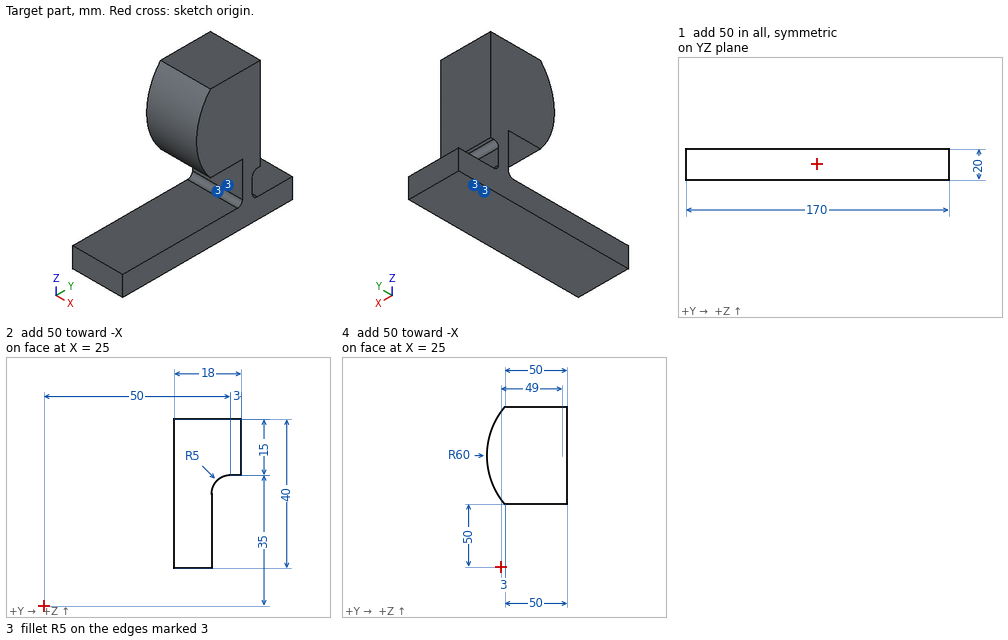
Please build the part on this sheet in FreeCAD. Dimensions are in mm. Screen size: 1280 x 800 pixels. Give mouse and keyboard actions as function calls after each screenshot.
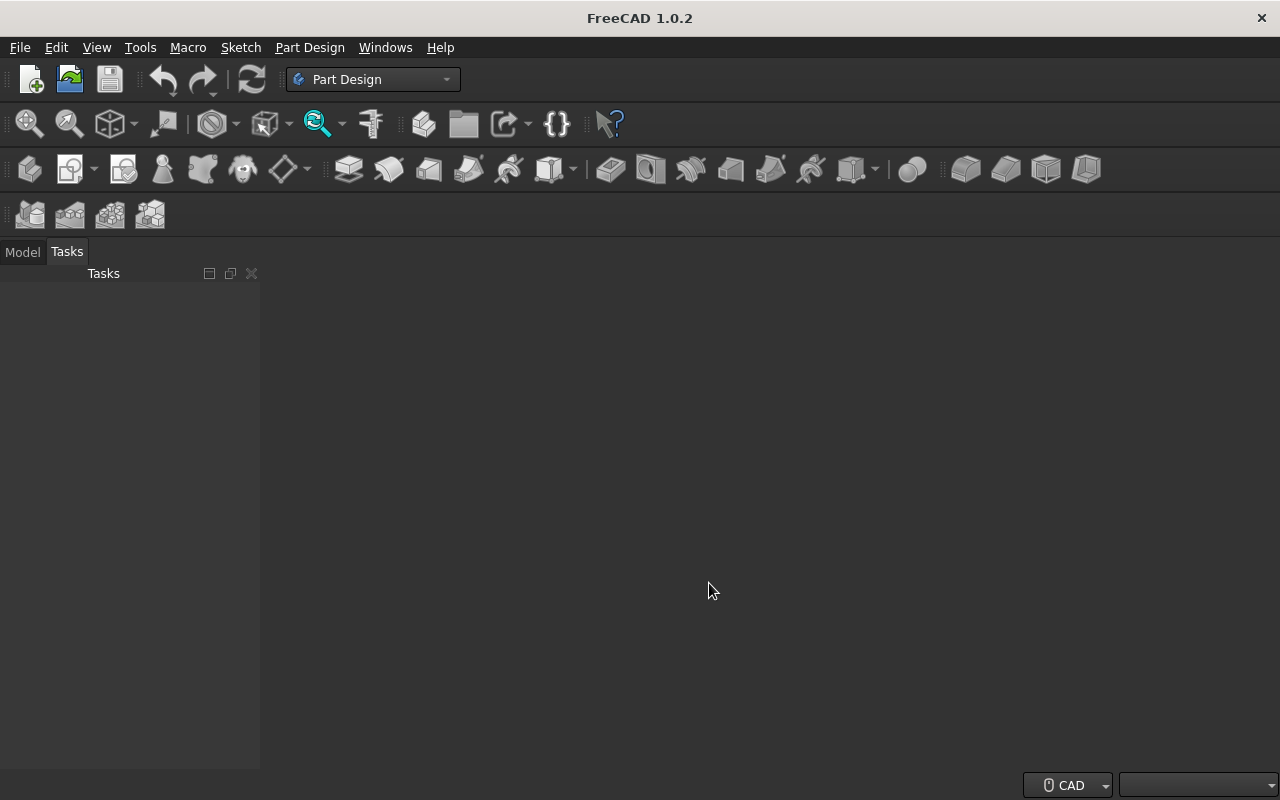
click(30, 80)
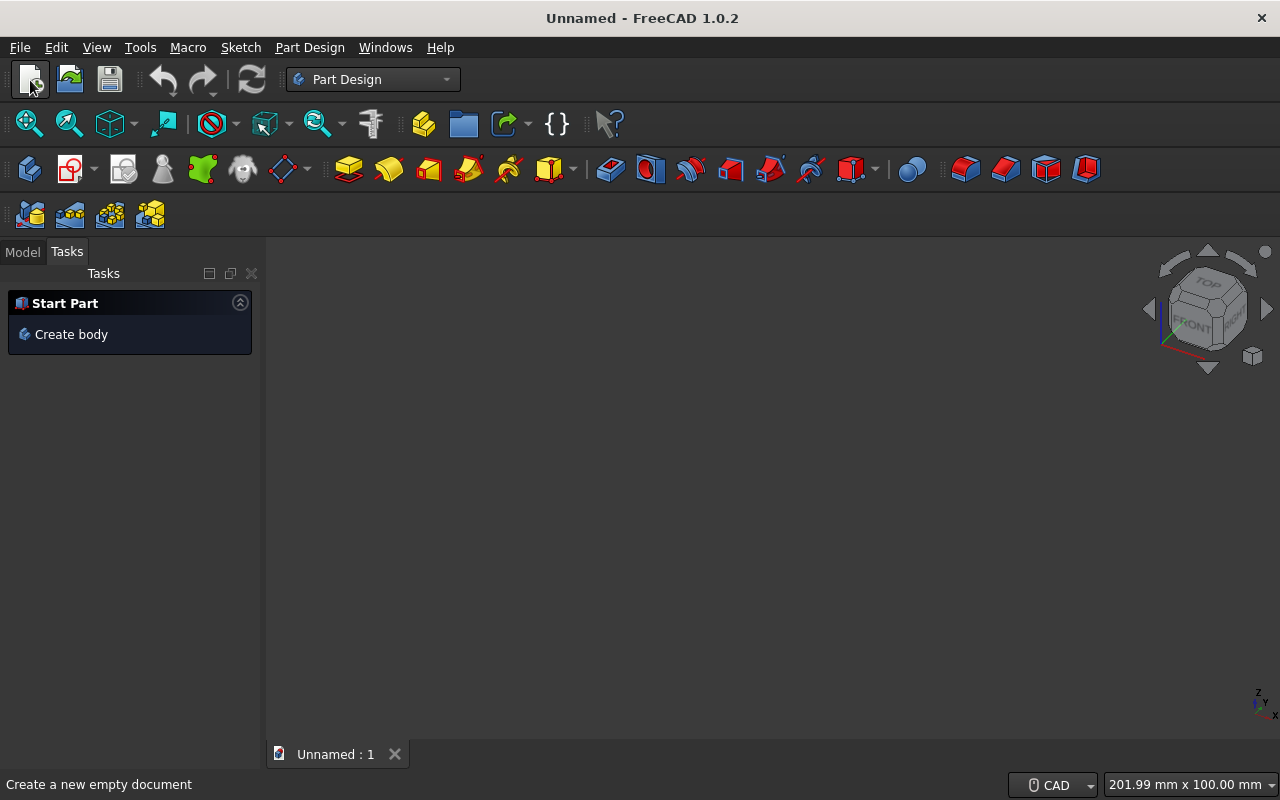
click(70, 170)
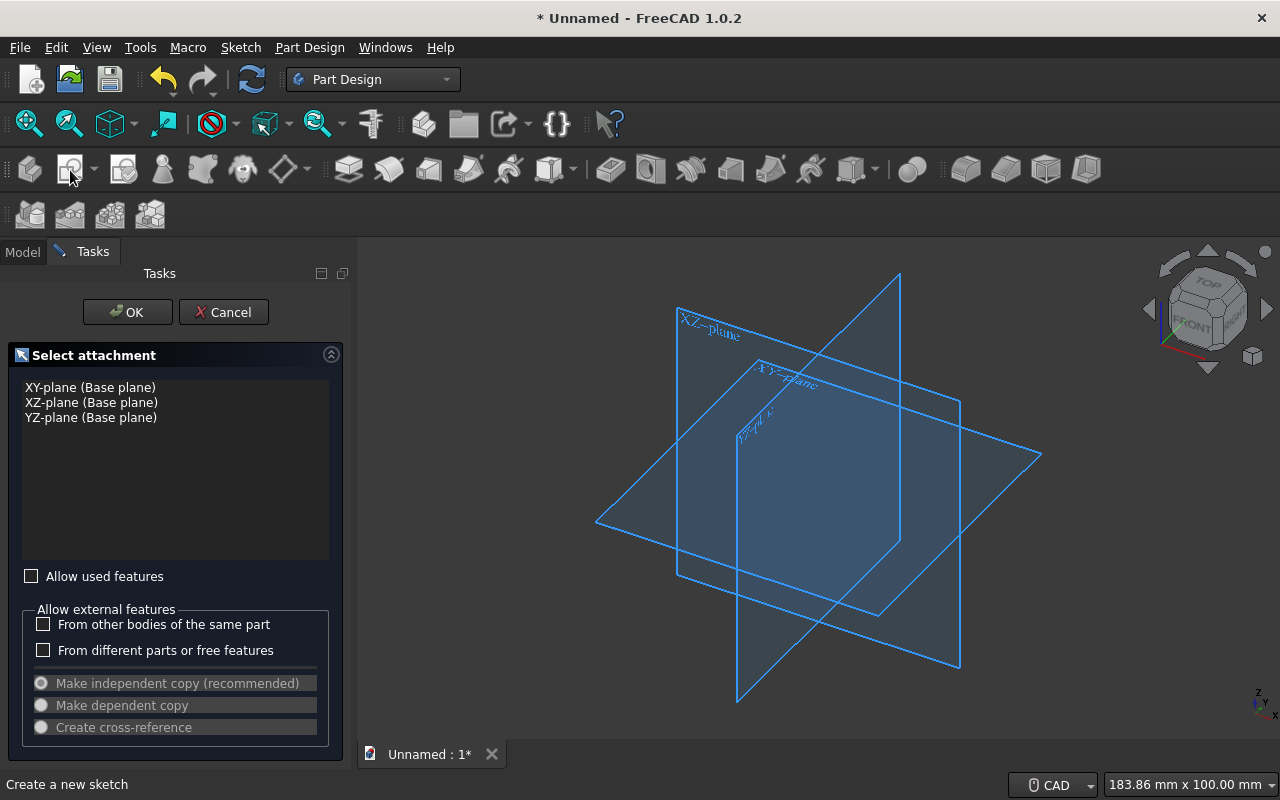
click(82, 418)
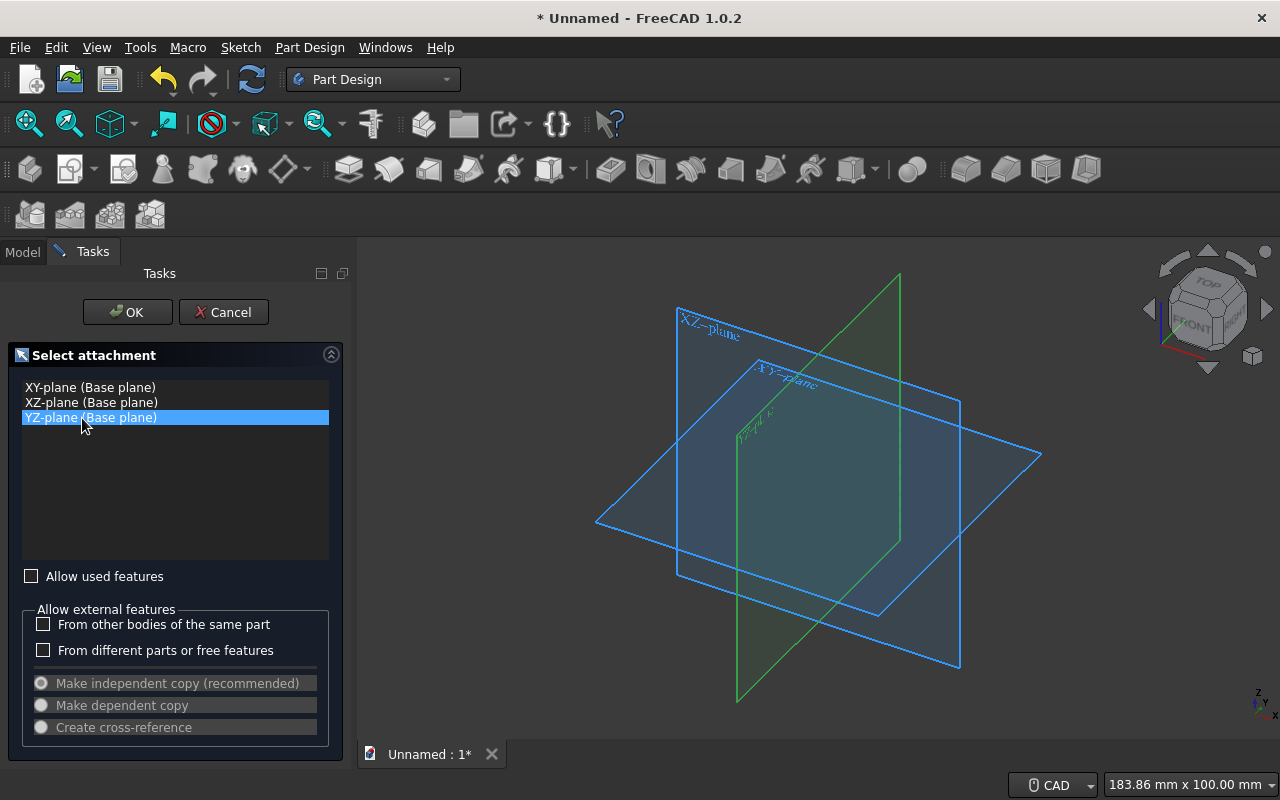
click(128, 312)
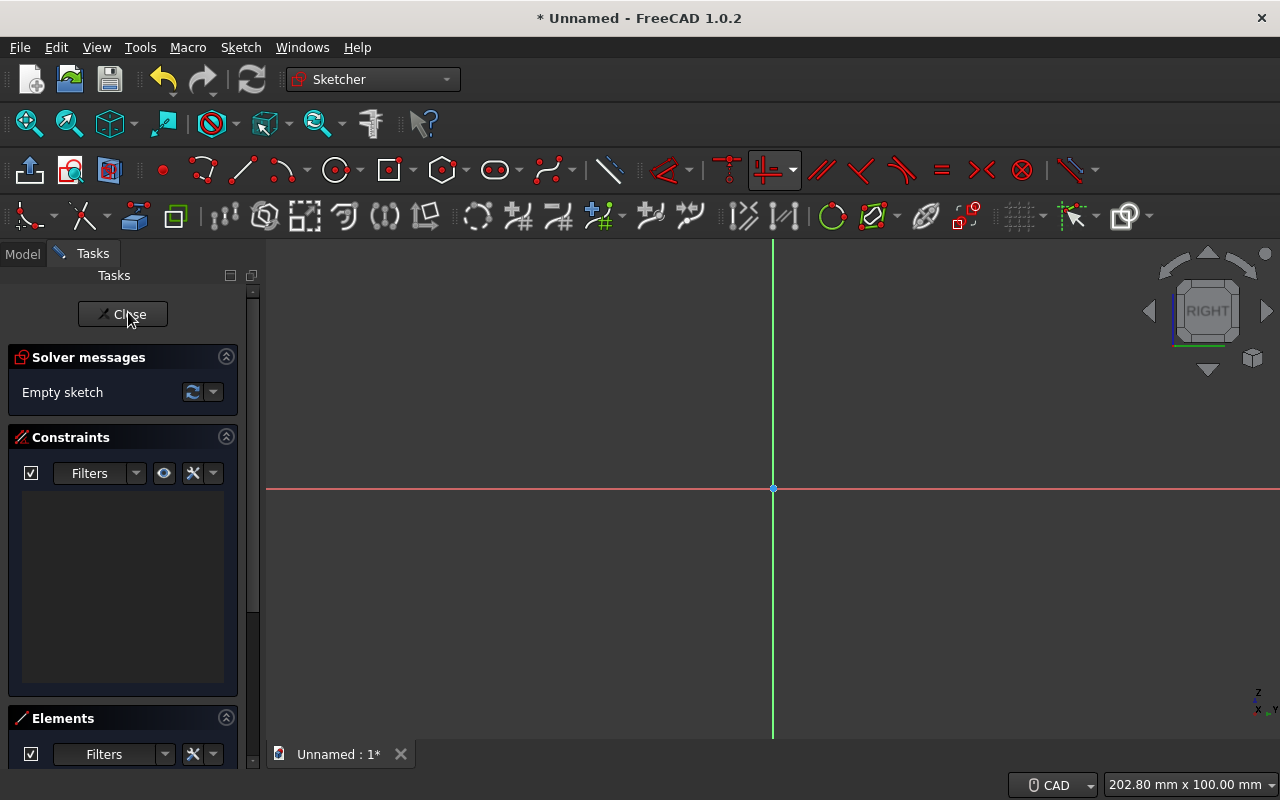
scroll(565, 489, down, 2)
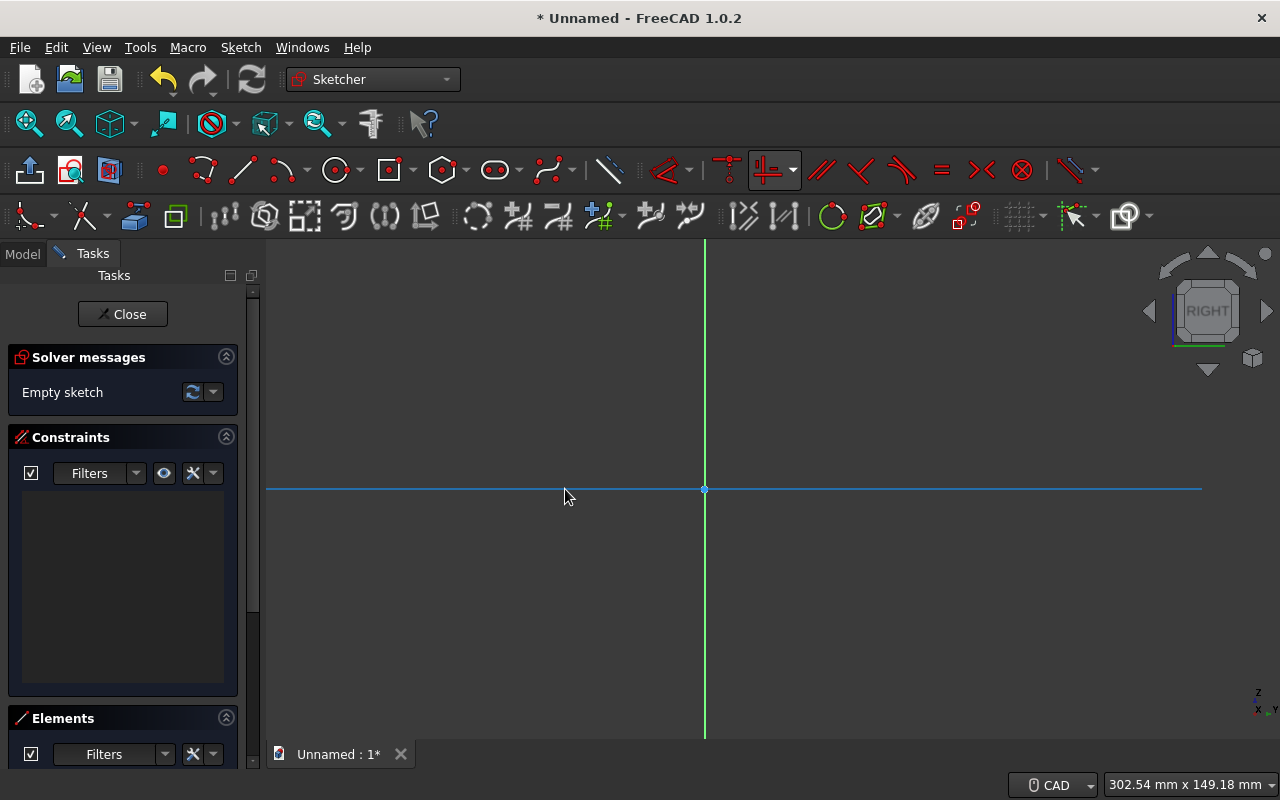
key(g)
key(v)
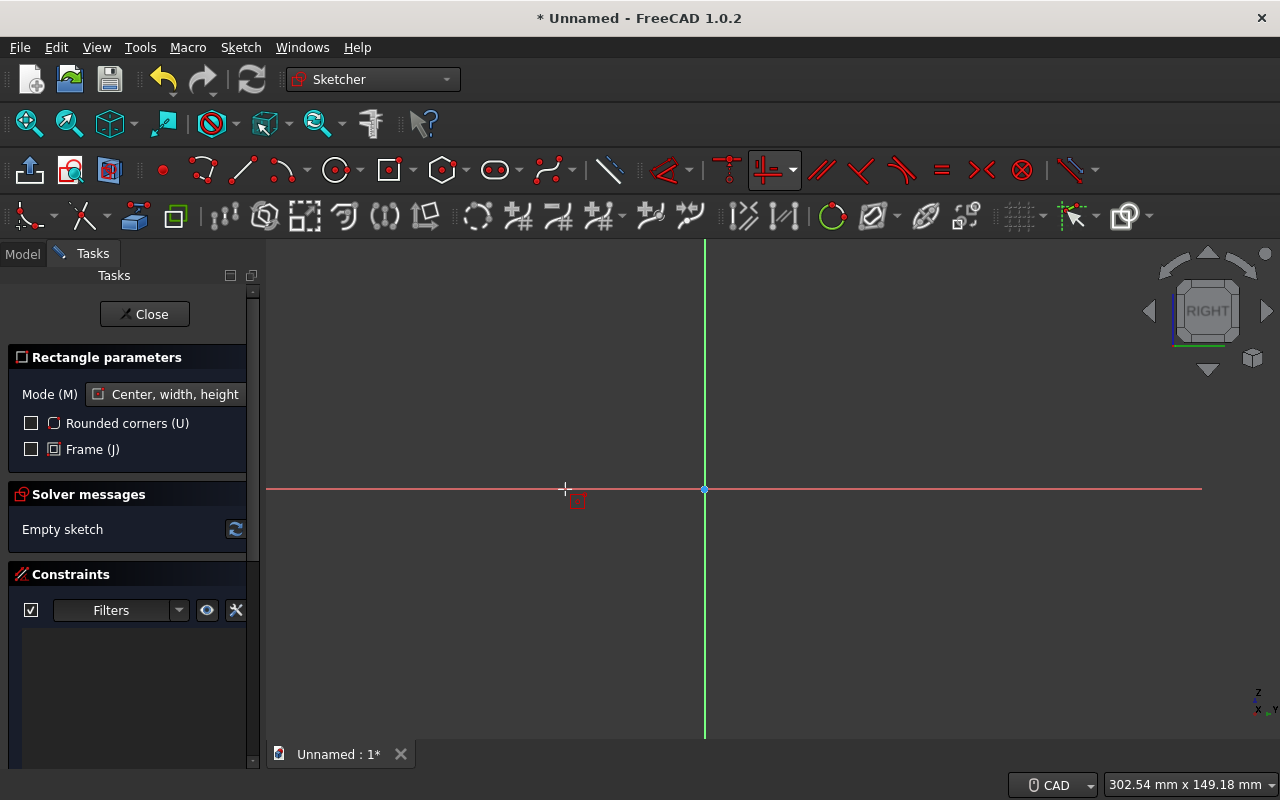
click(705, 489)
click(989, 456)
key(Escape)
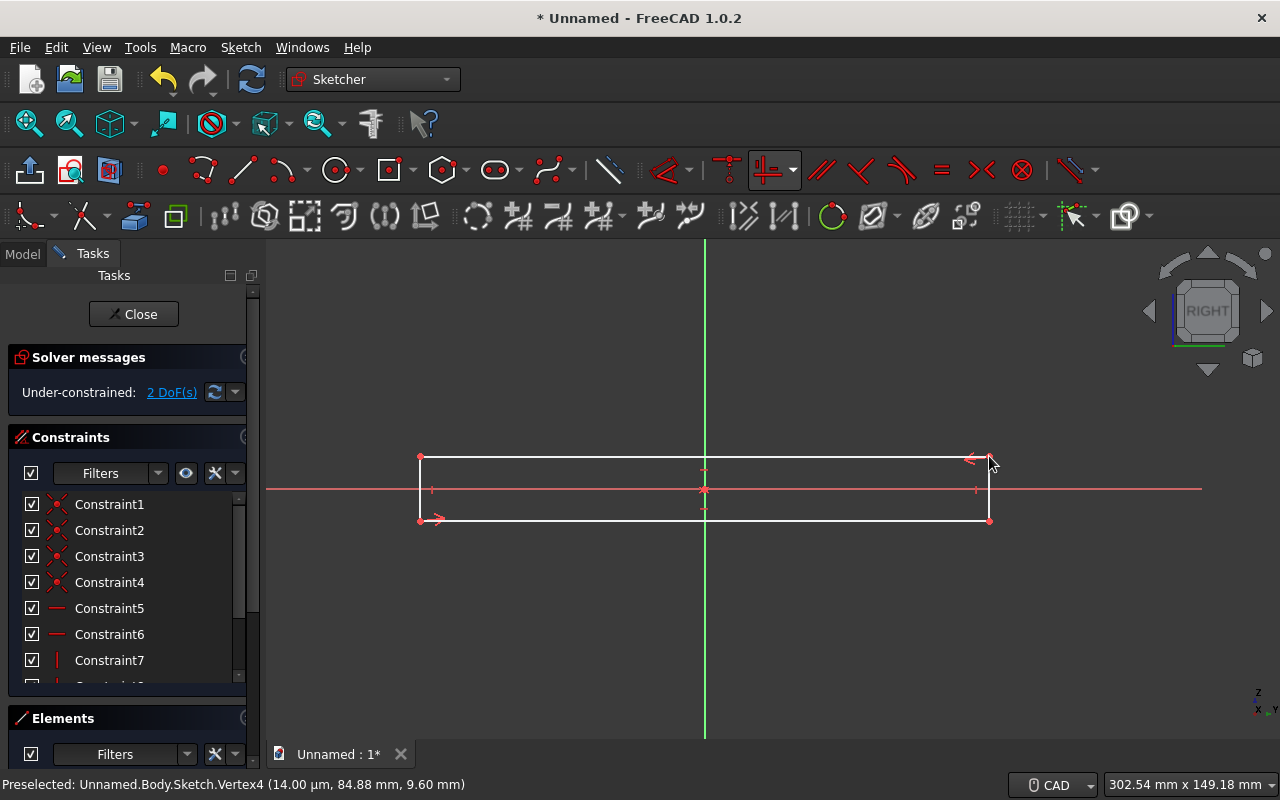
key(d)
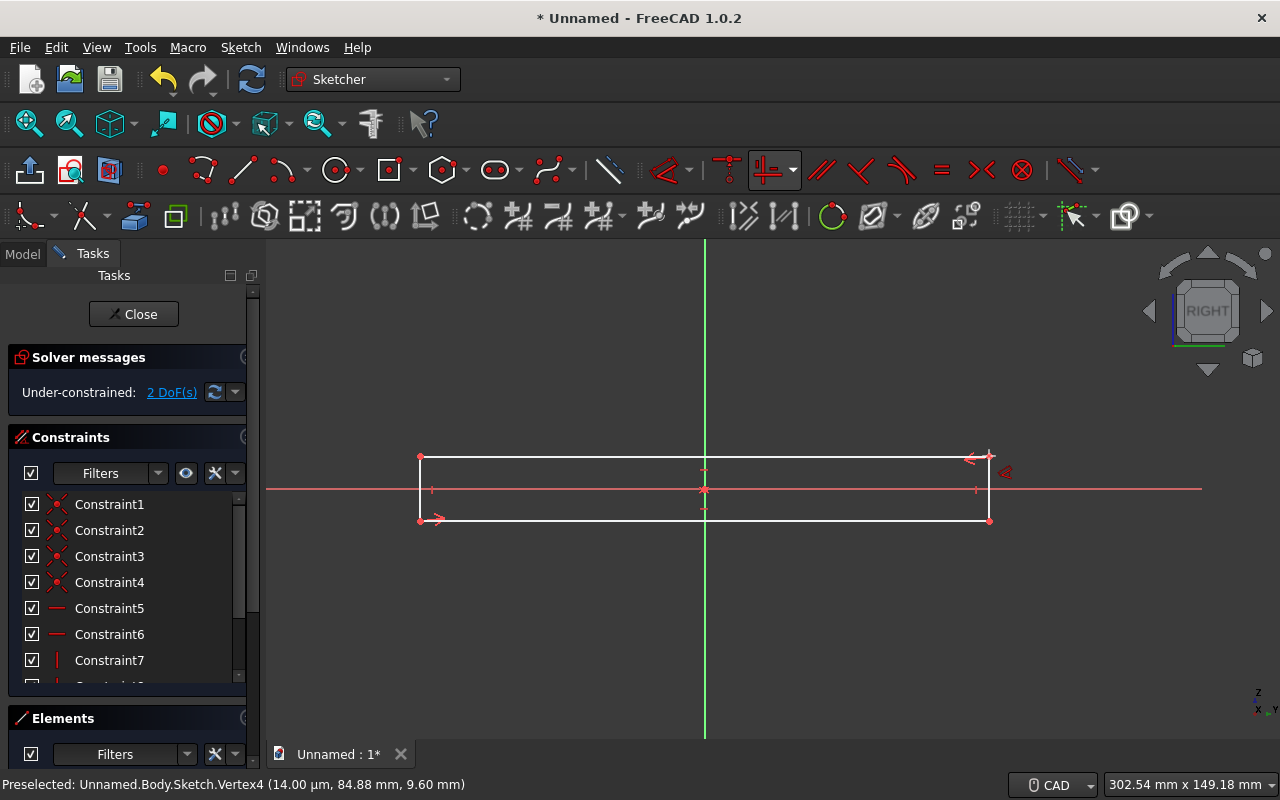
click(989, 502)
click(1023, 474)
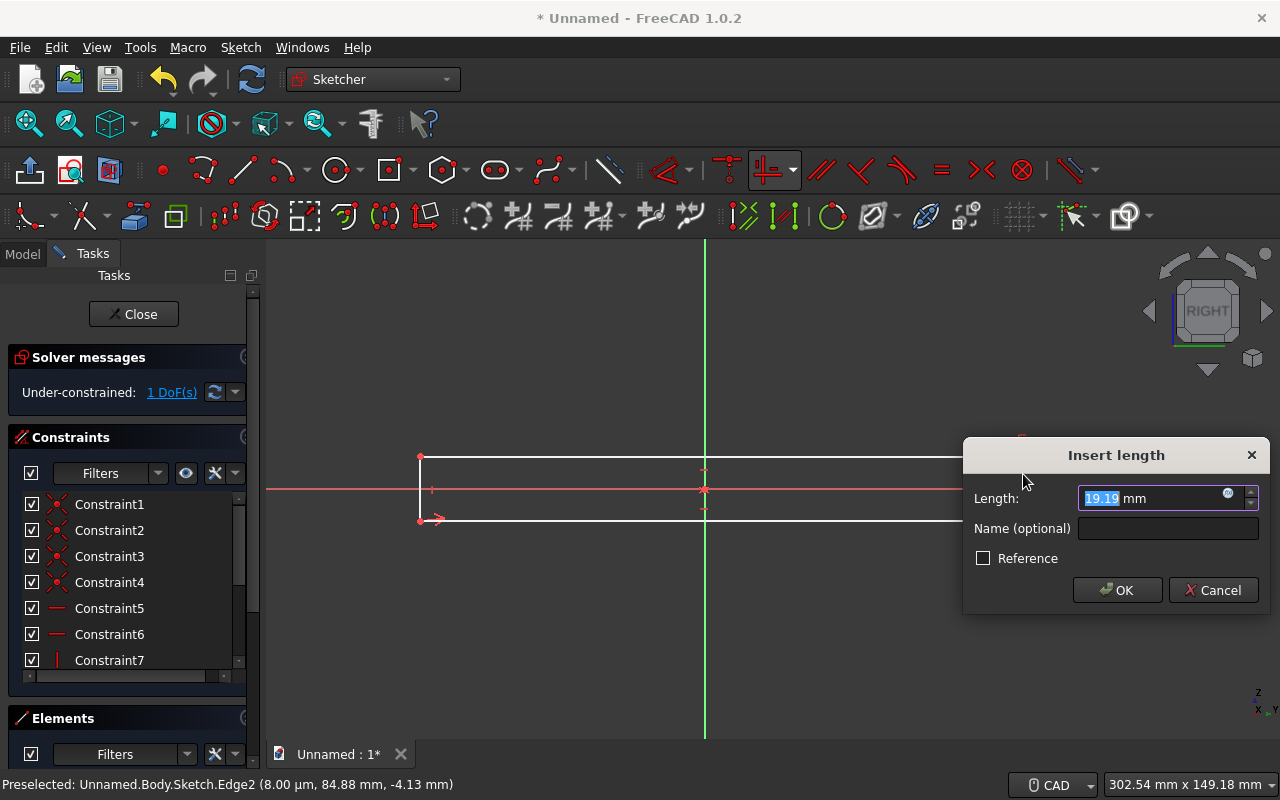
text(20)
key(Return)